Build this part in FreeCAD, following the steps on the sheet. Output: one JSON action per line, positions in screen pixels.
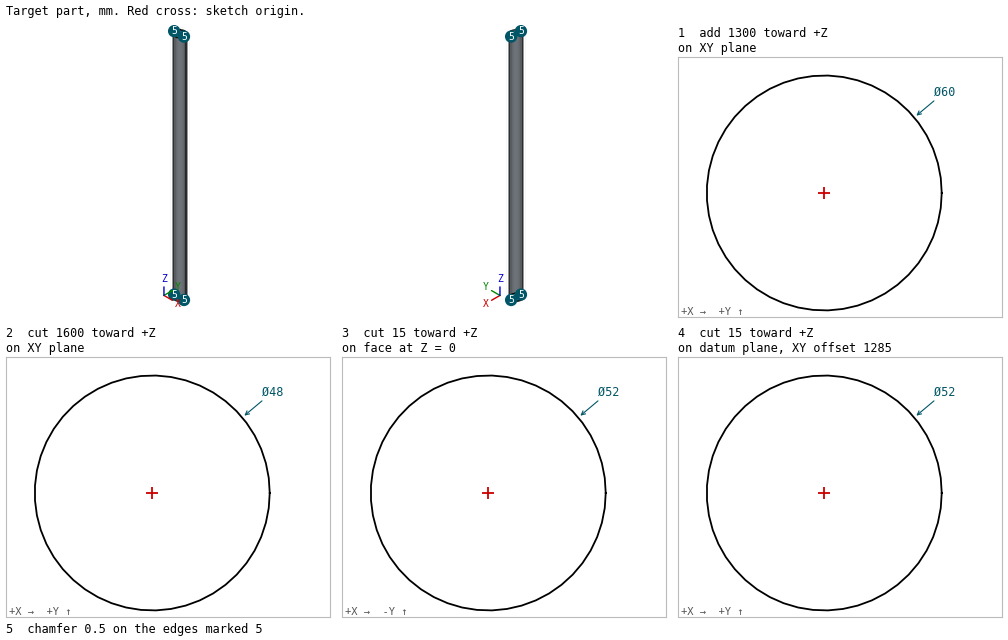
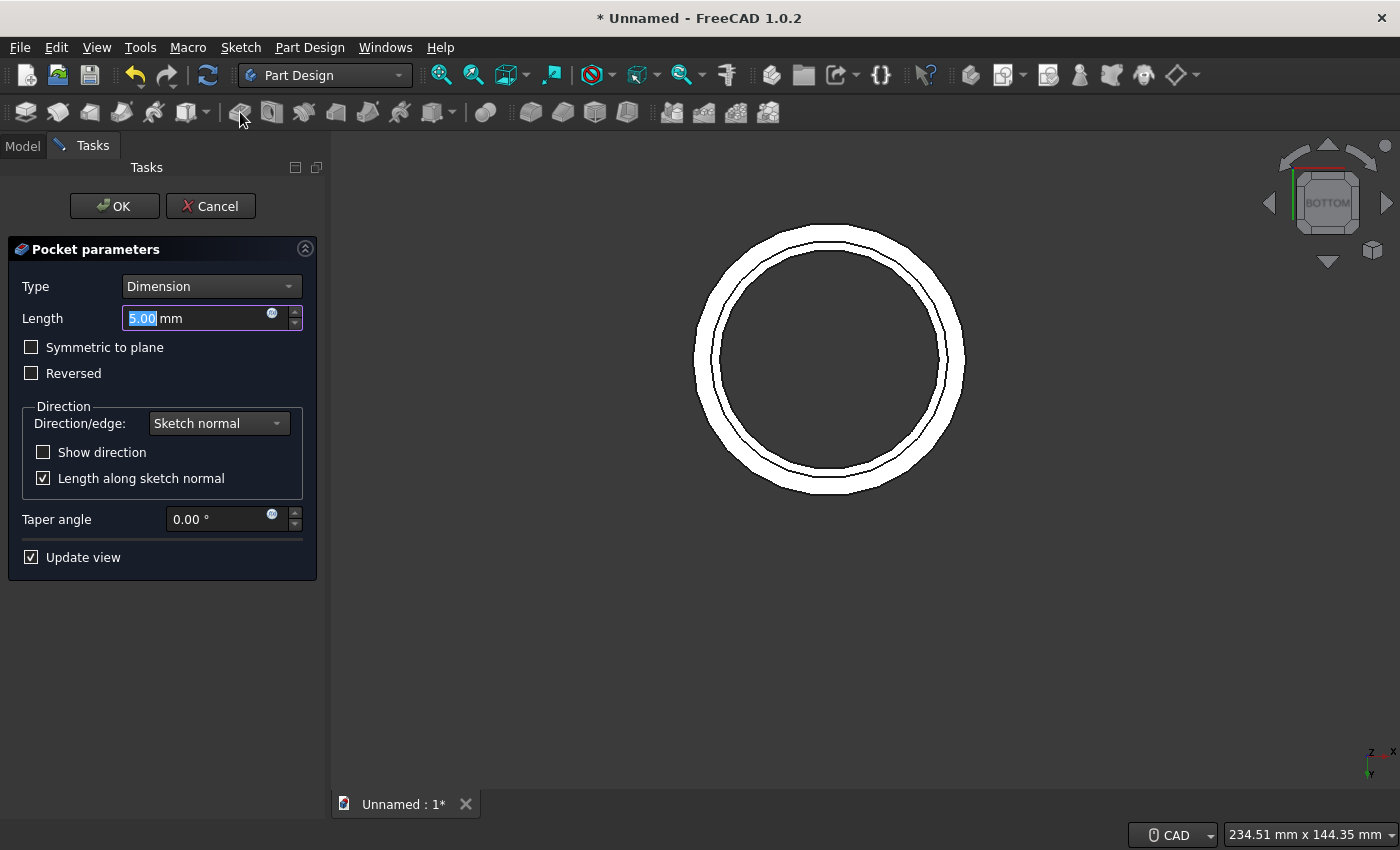
{"action": "type", "text": "15"}
{"action": "key", "text": "Tab"}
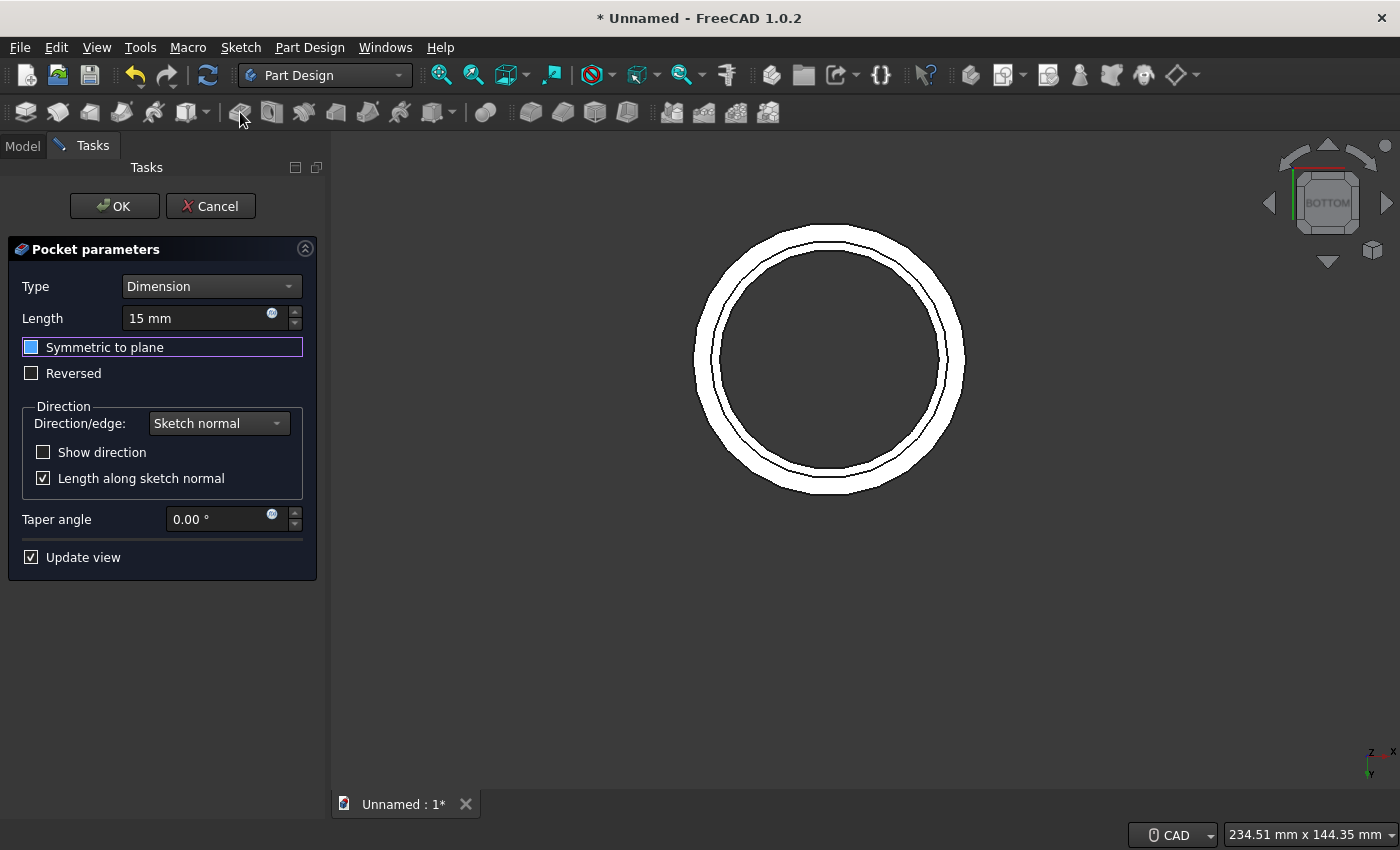
{"action": "left_click", "coordinate": [115, 206]}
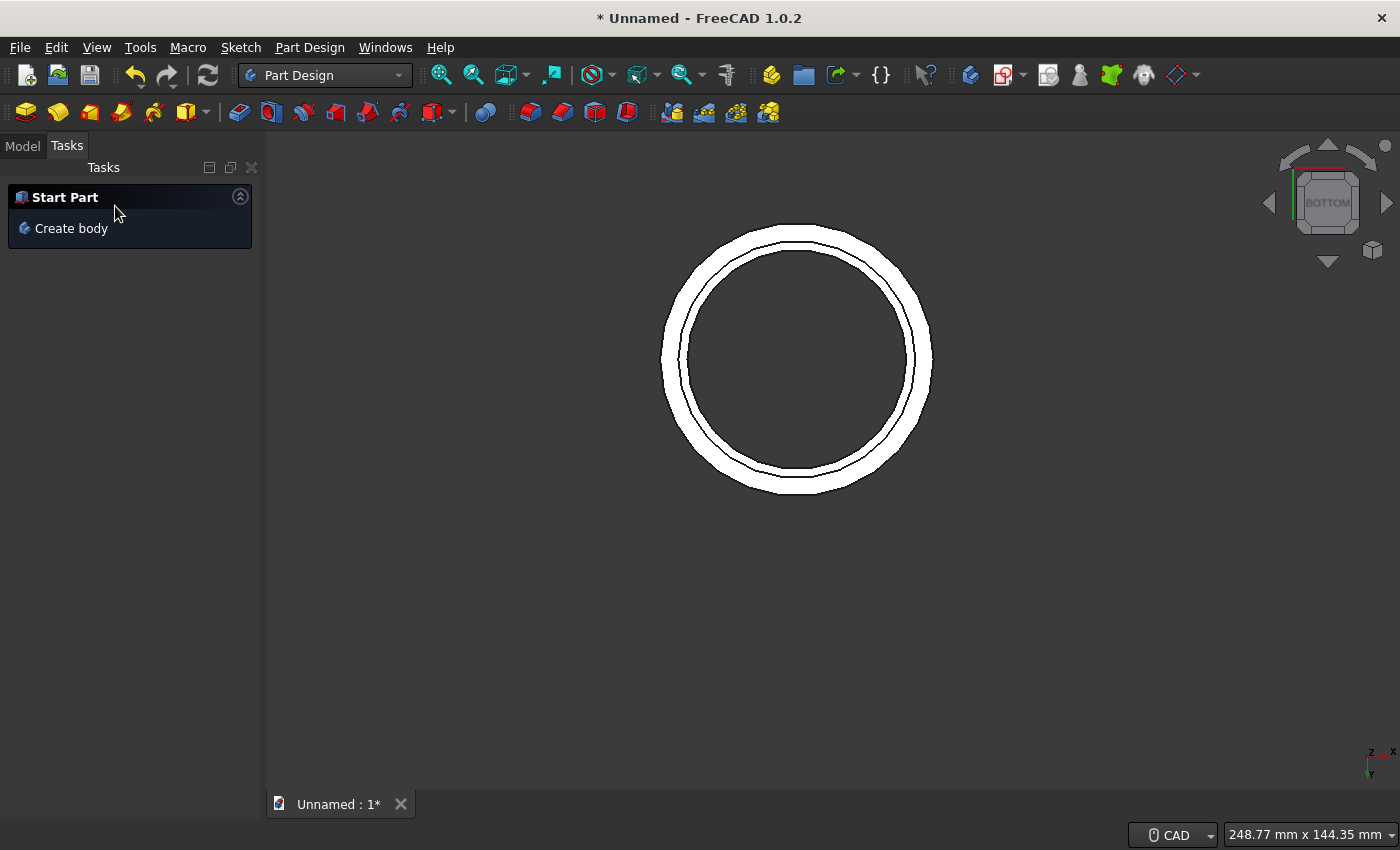
{"action": "left_click", "coordinate": [442, 76]}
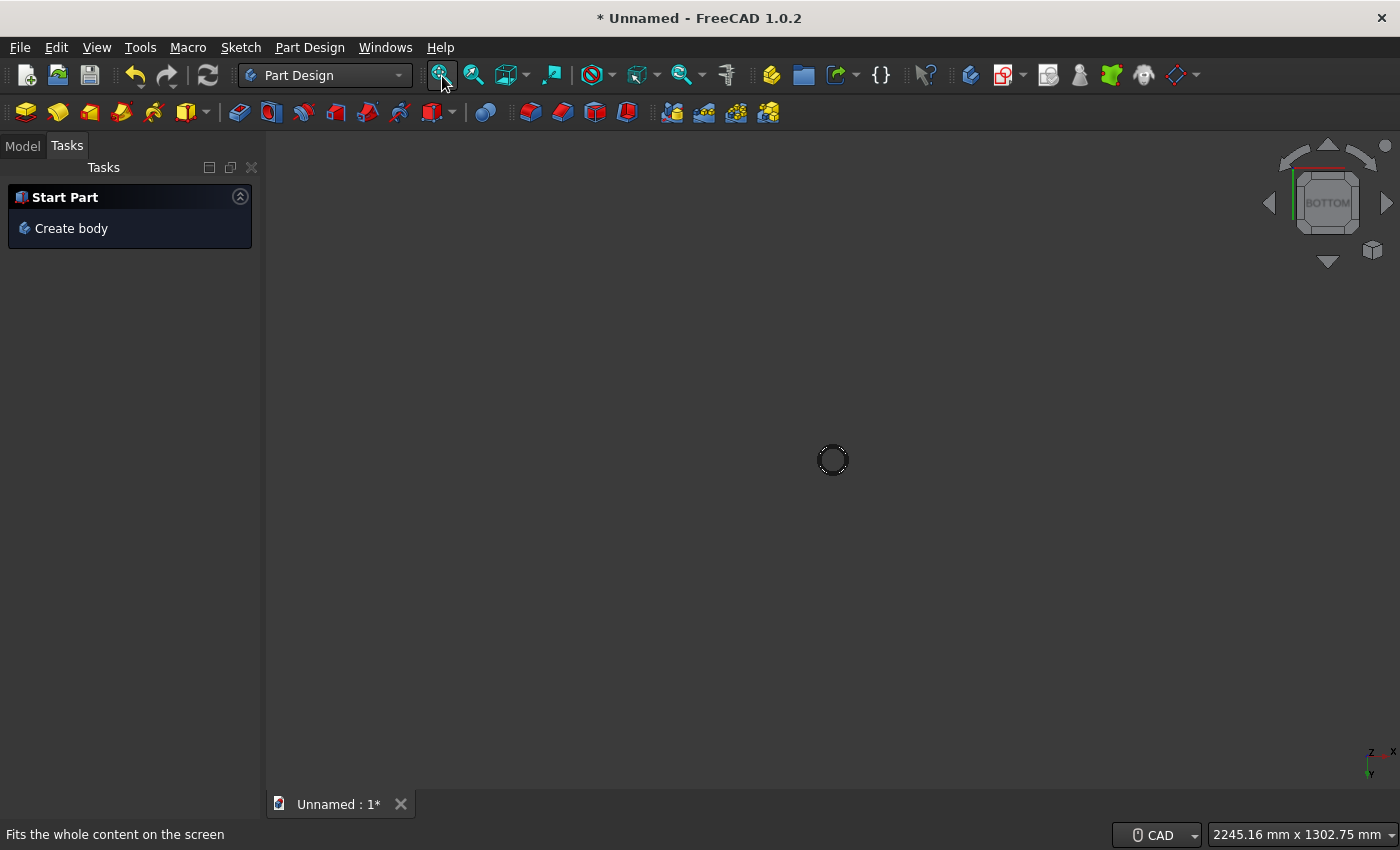
{"action": "left_click", "coordinate": [23, 145]}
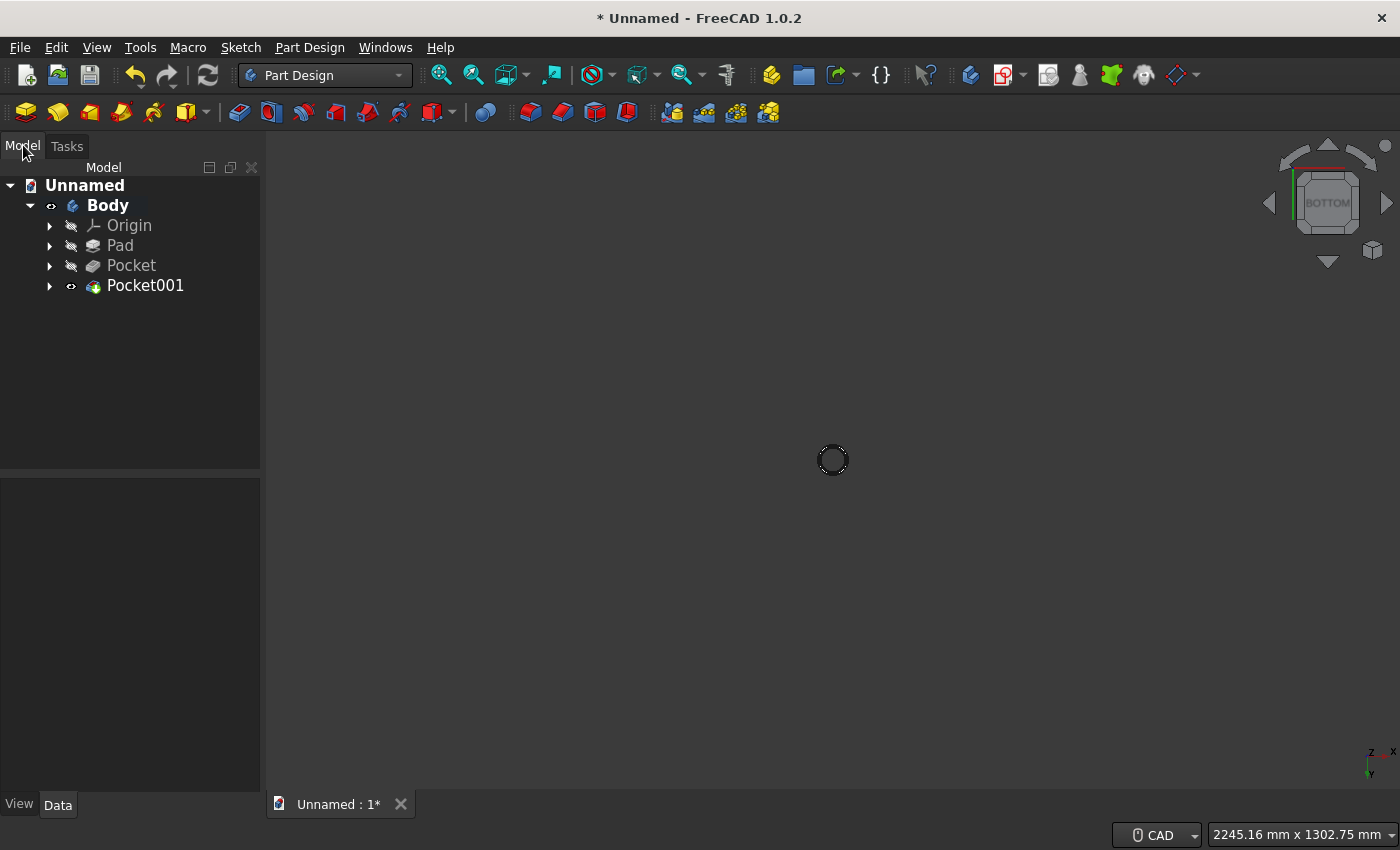
{"action": "left_click", "coordinate": [50, 226]}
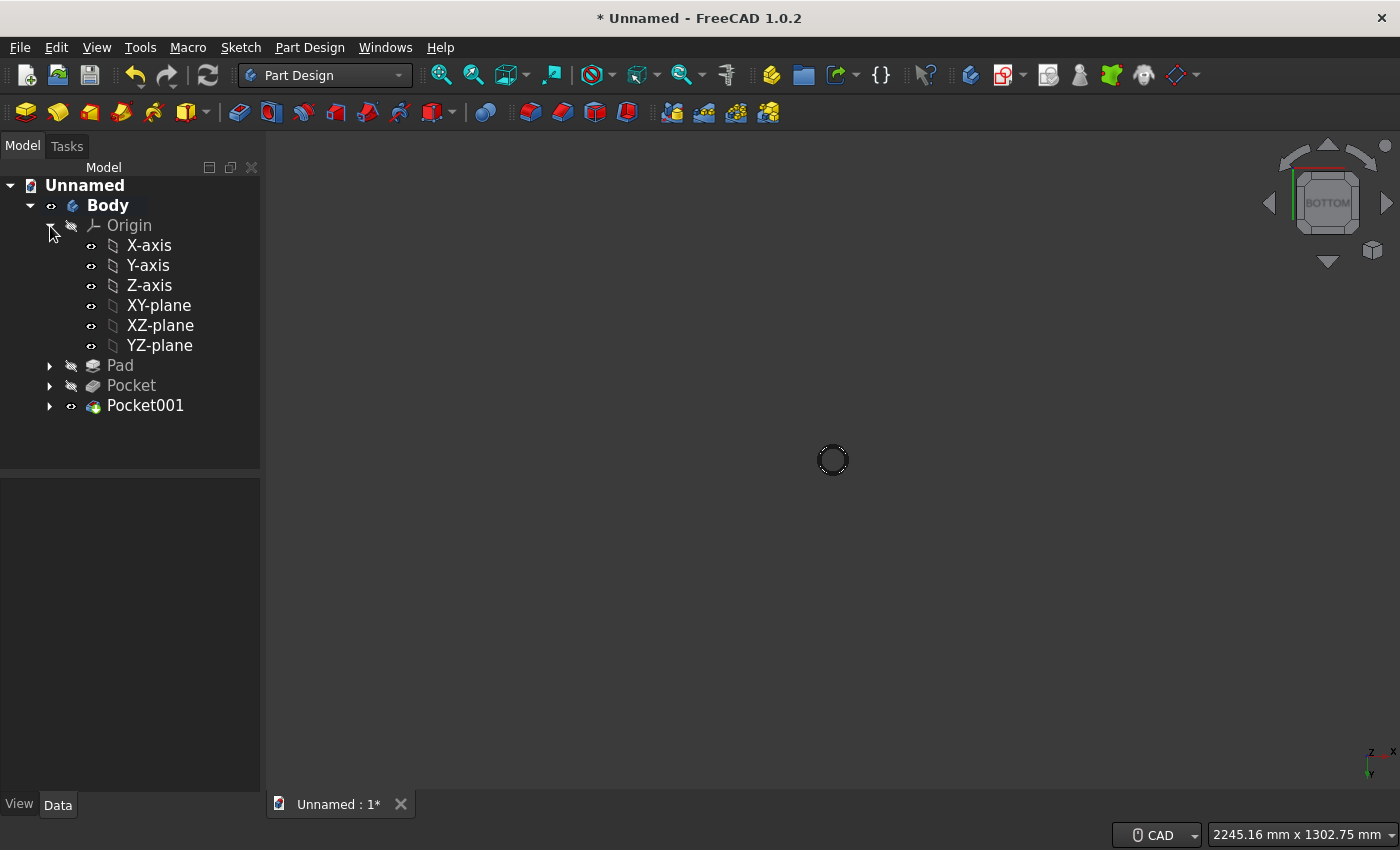
{"action": "left_click", "coordinate": [136, 306]}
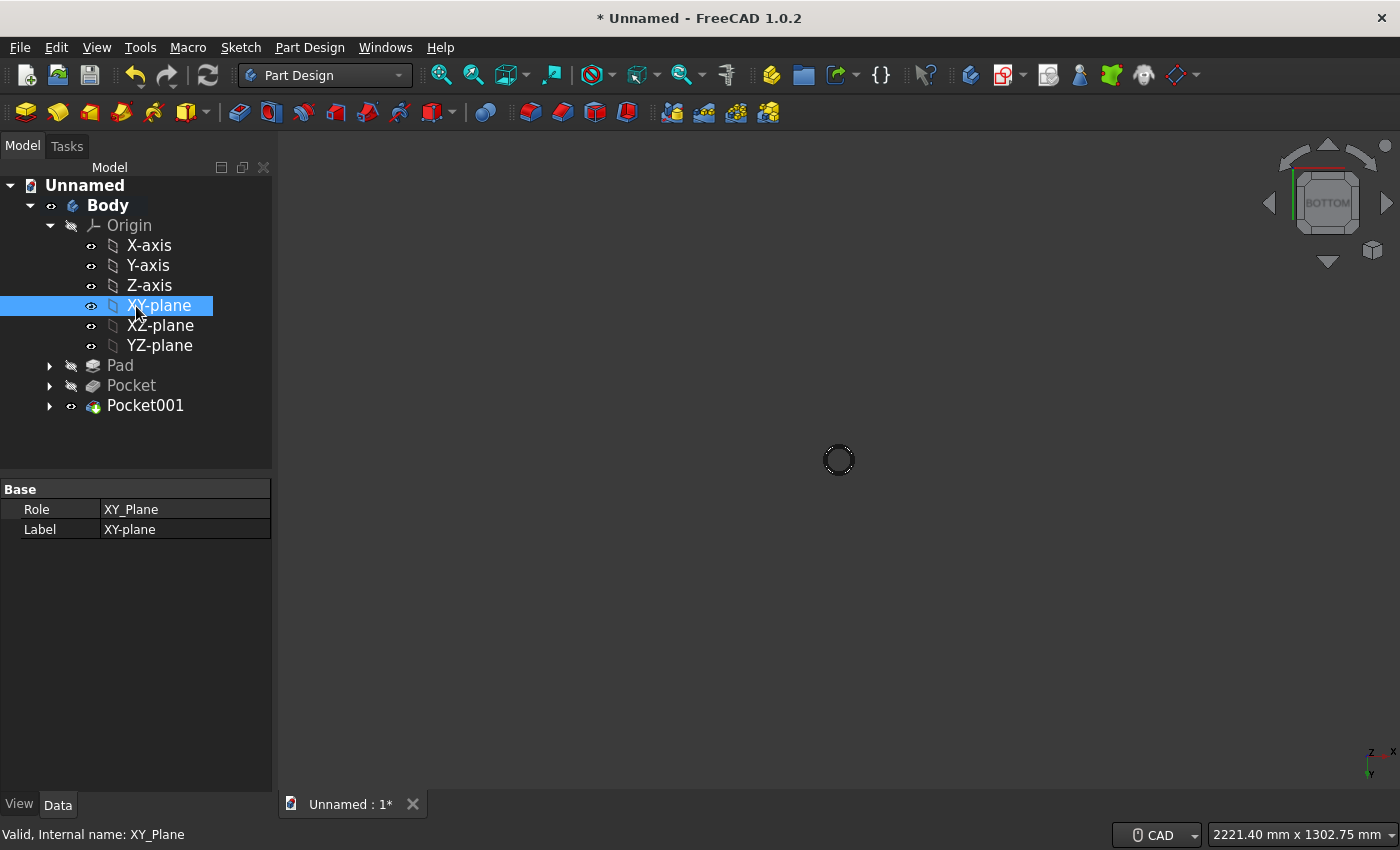
{"action": "left_click", "coordinate": [1176, 76]}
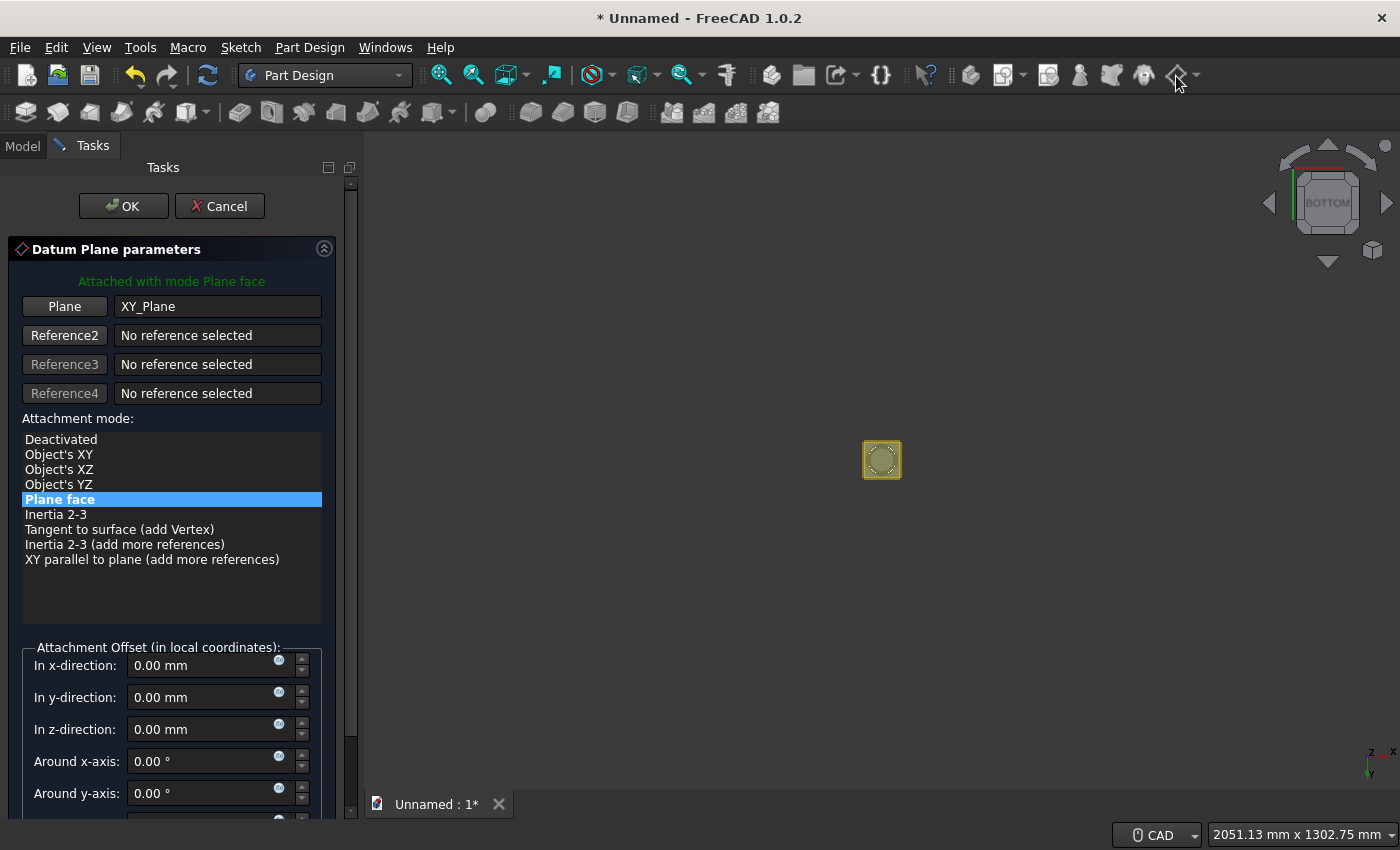
{"action": "triple_click", "coordinate": [210, 729]}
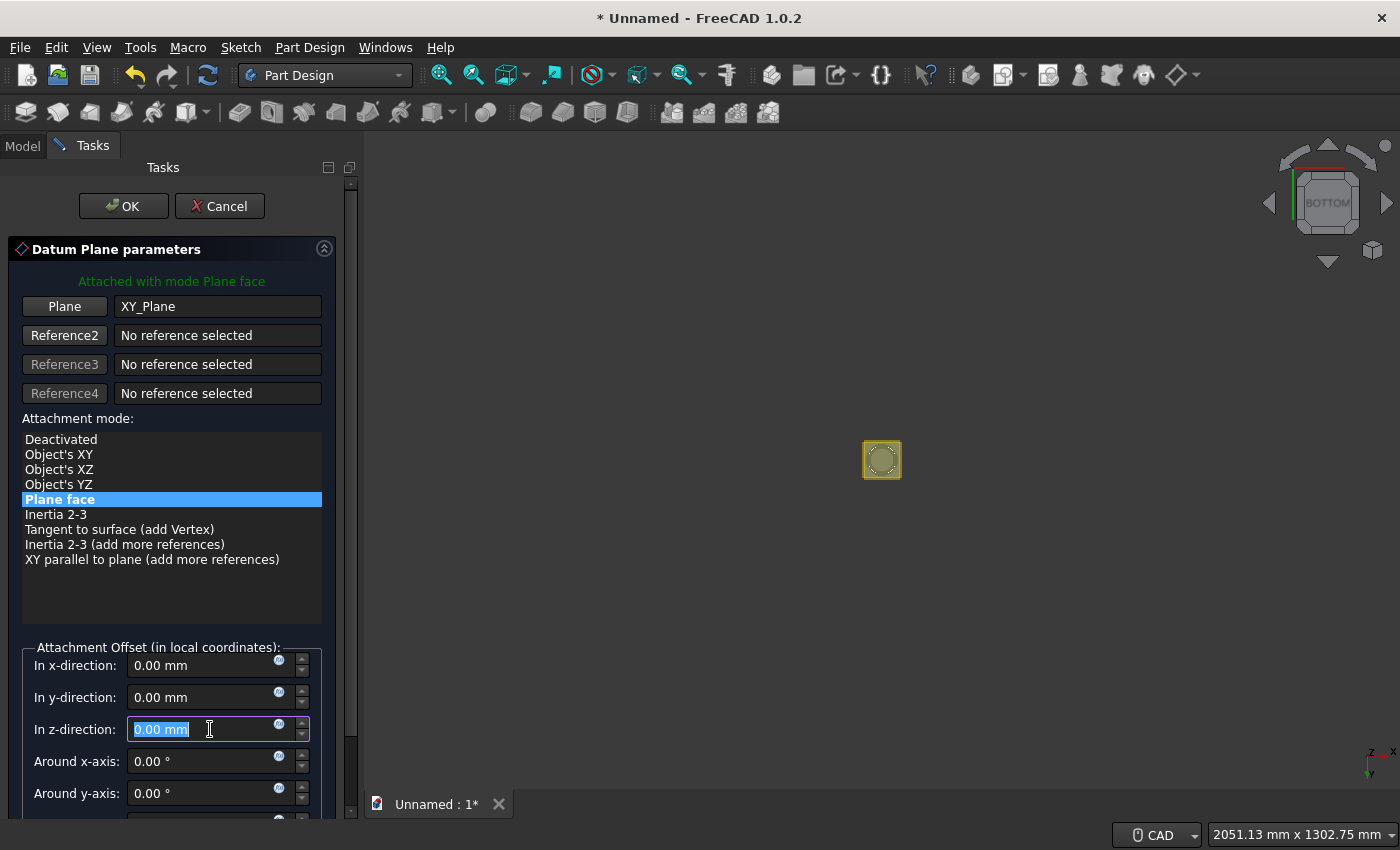
{"action": "type", "text": "1285"}
{"action": "key", "text": "Tab"}